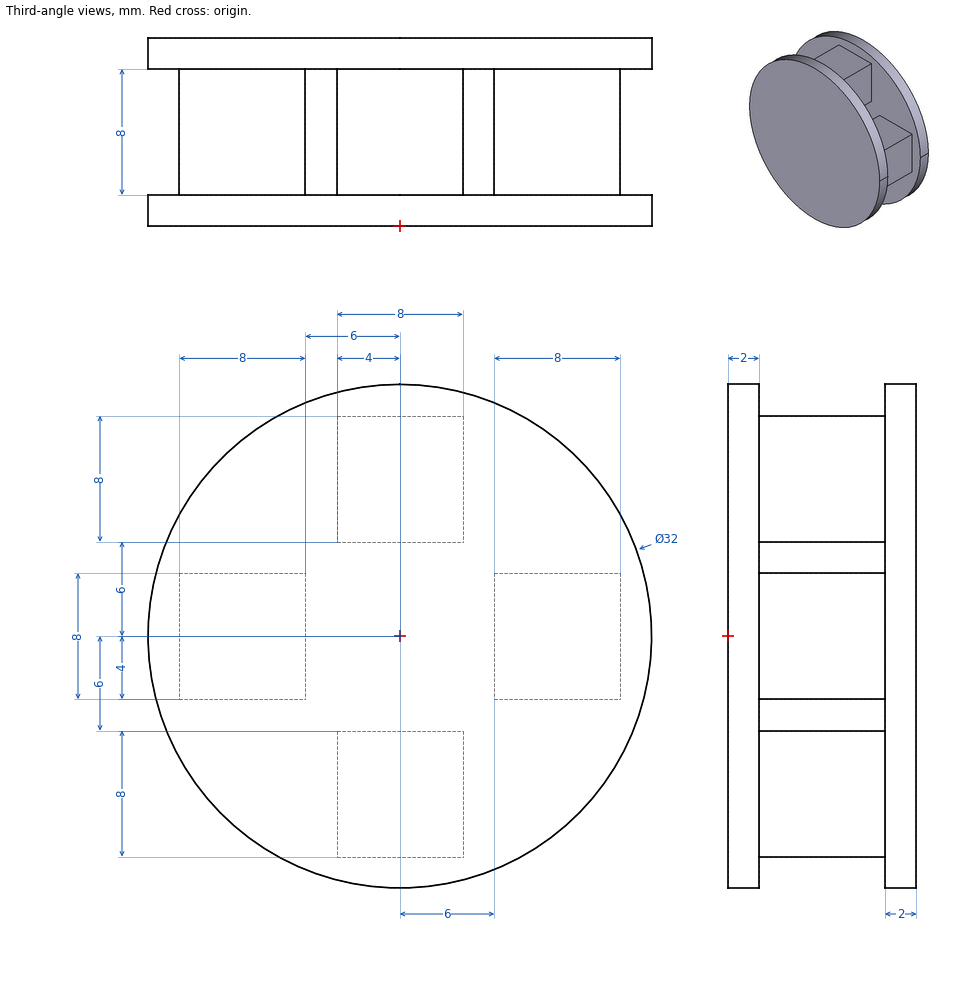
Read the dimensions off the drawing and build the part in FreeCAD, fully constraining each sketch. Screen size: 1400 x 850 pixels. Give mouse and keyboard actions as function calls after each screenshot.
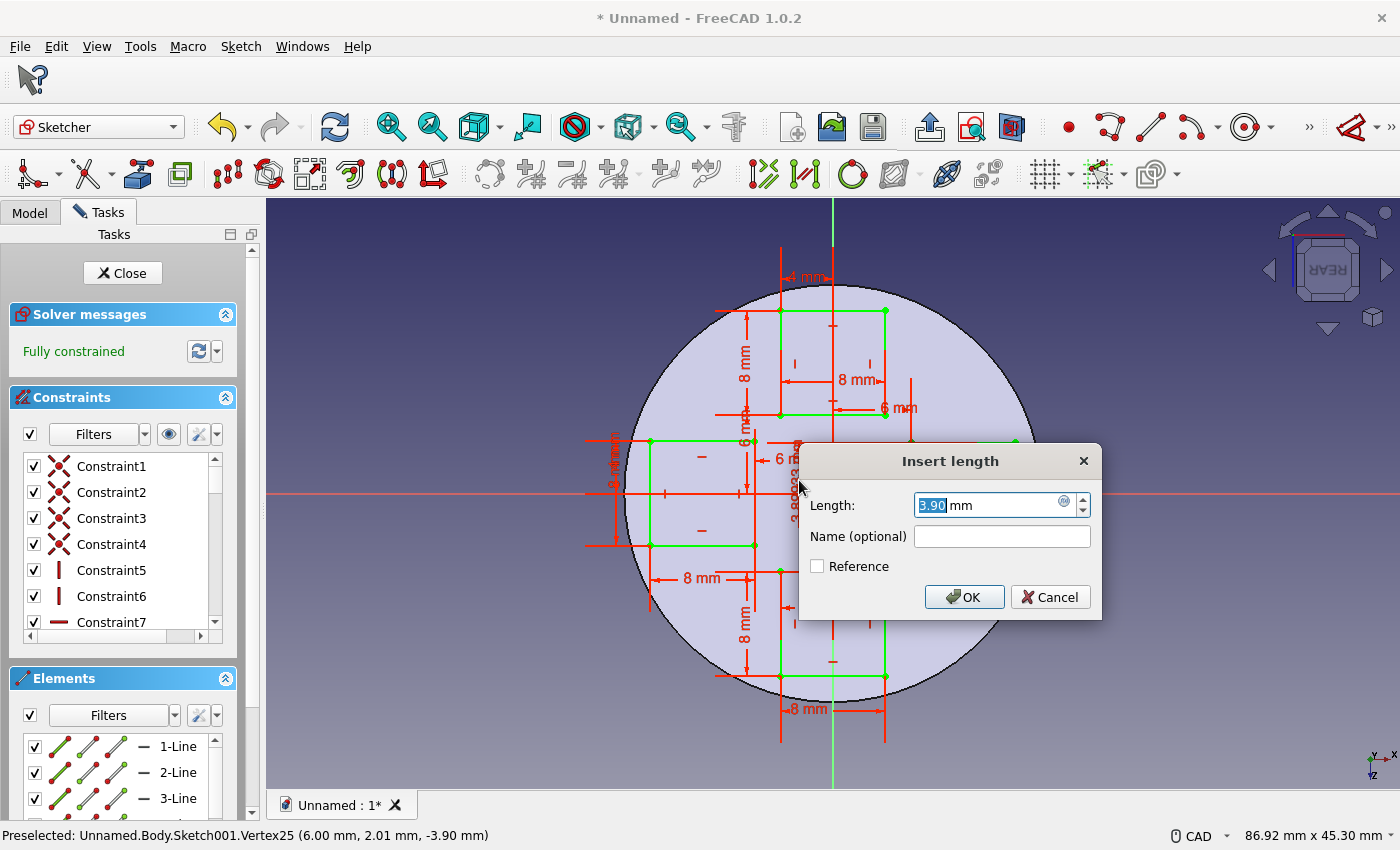
text(4)
key(Return)
key(Escape)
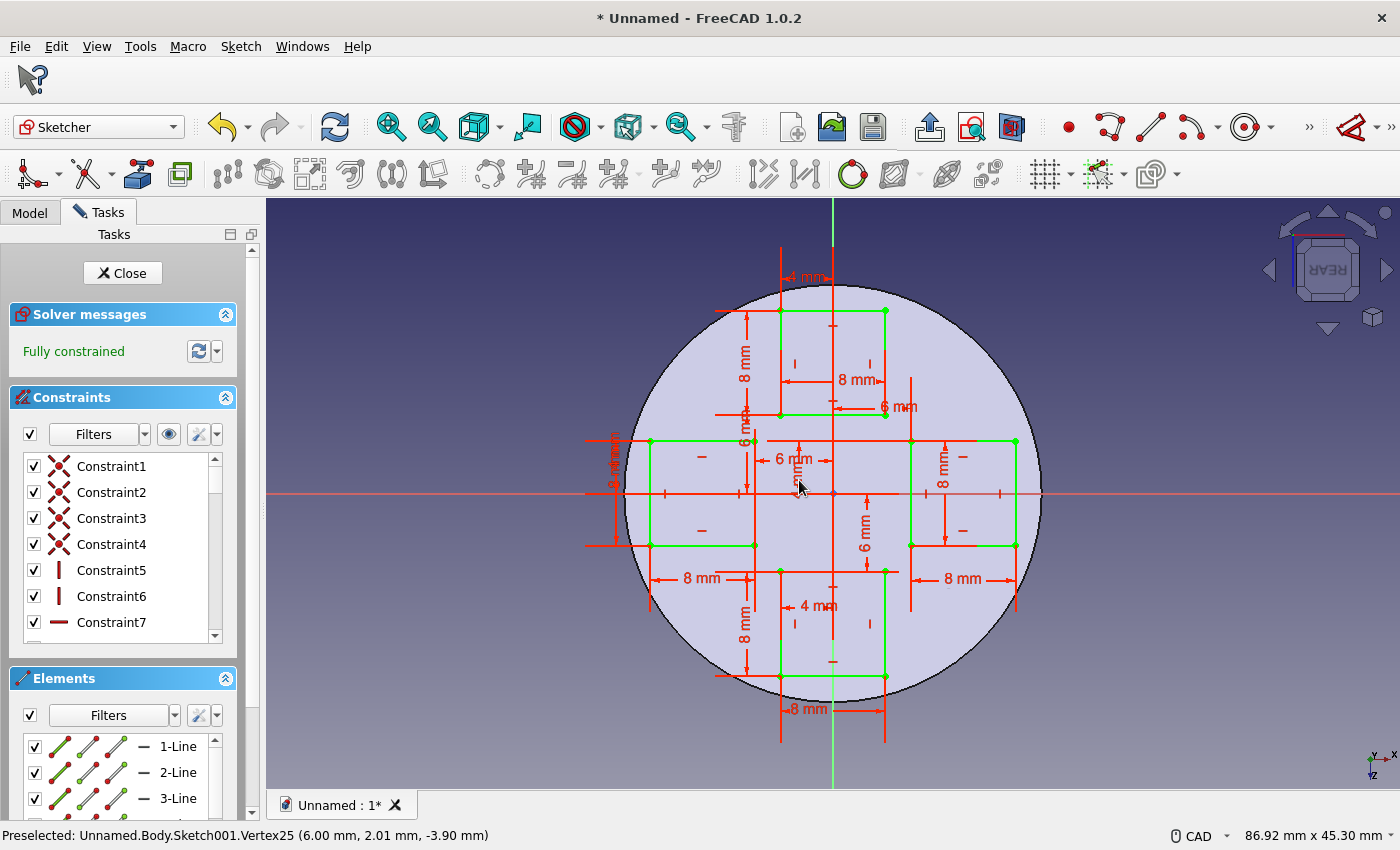
click(123, 273)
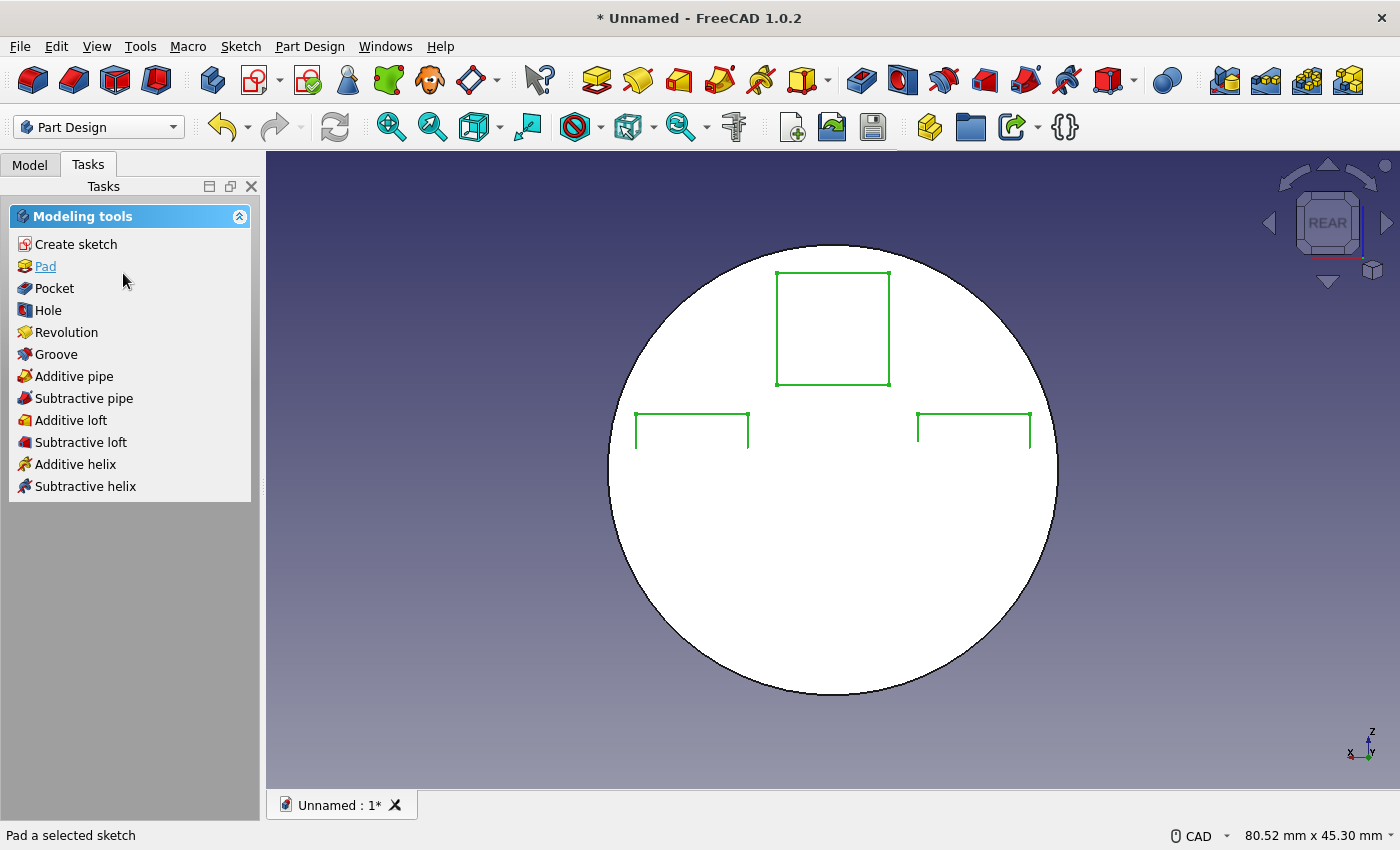
click(597, 80)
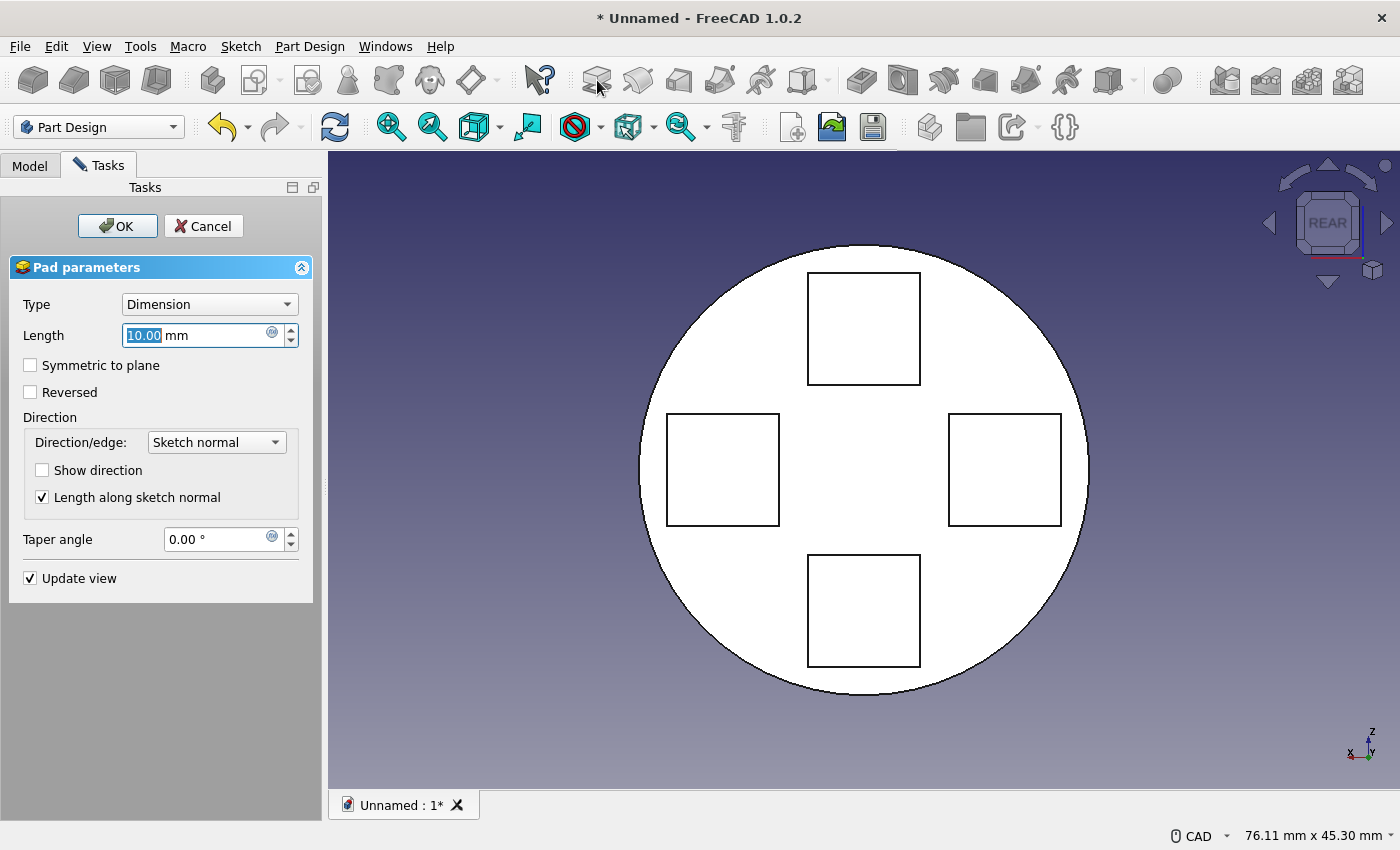
text(8)
key(Tab)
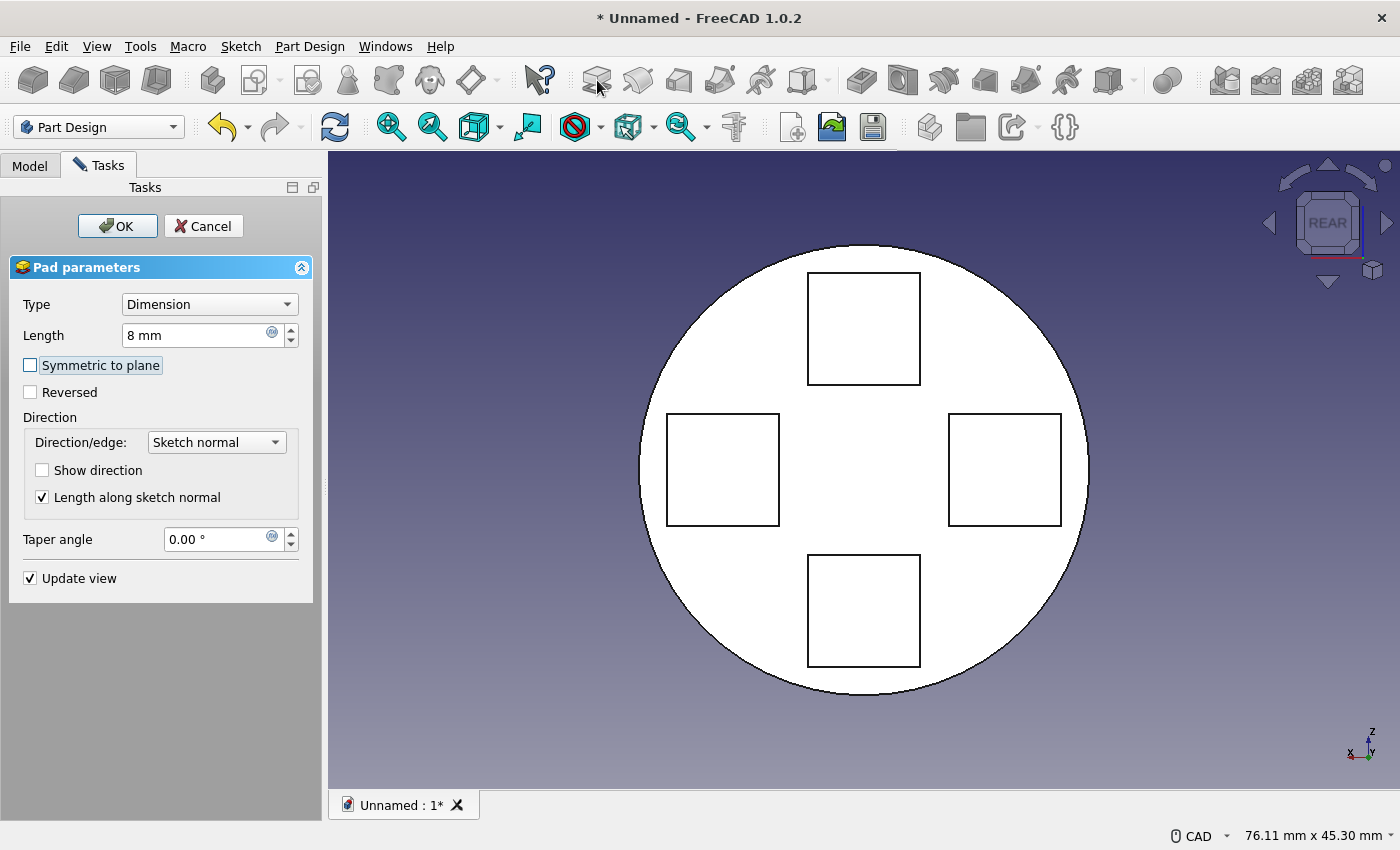
click(118, 226)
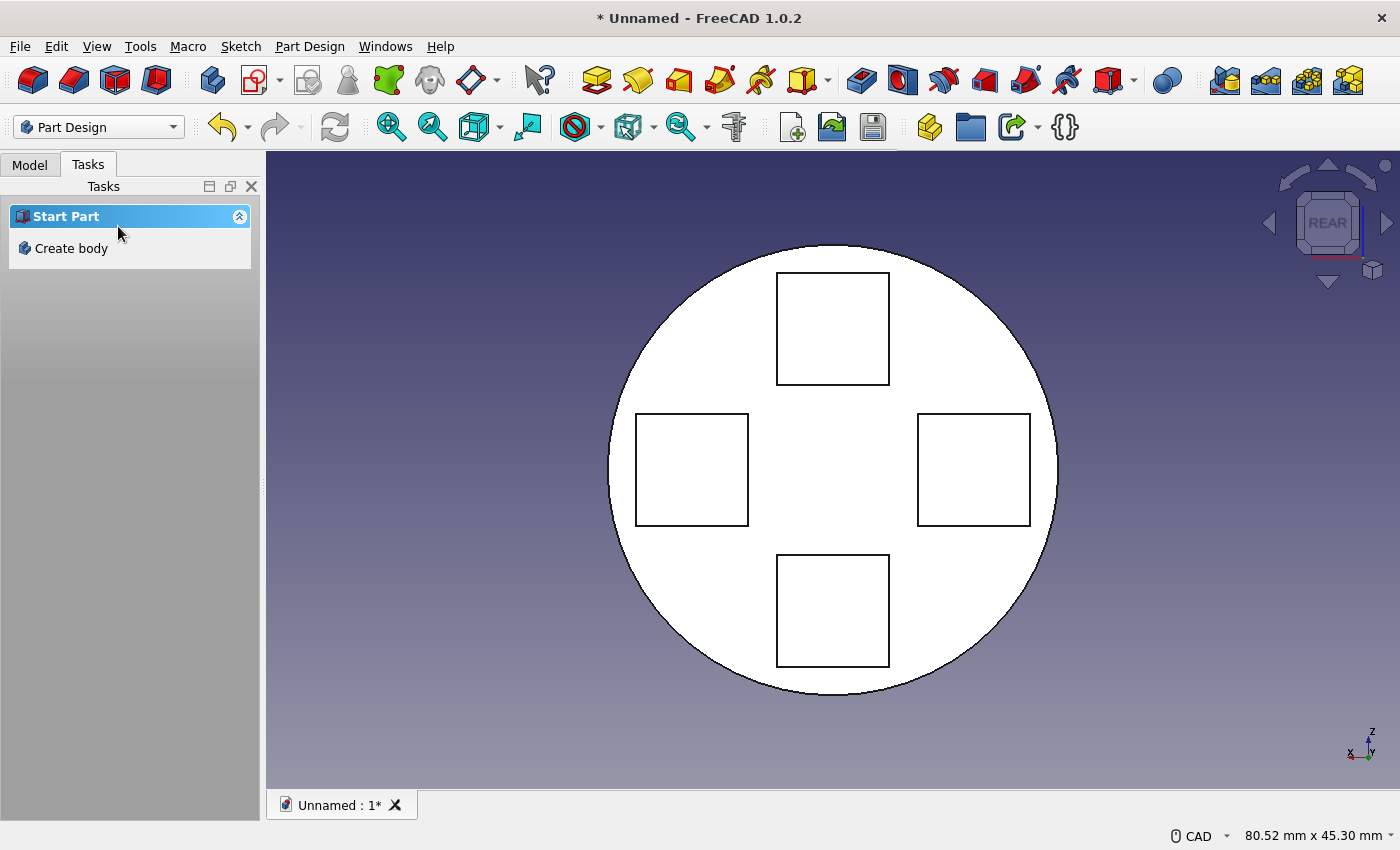
click(692, 469)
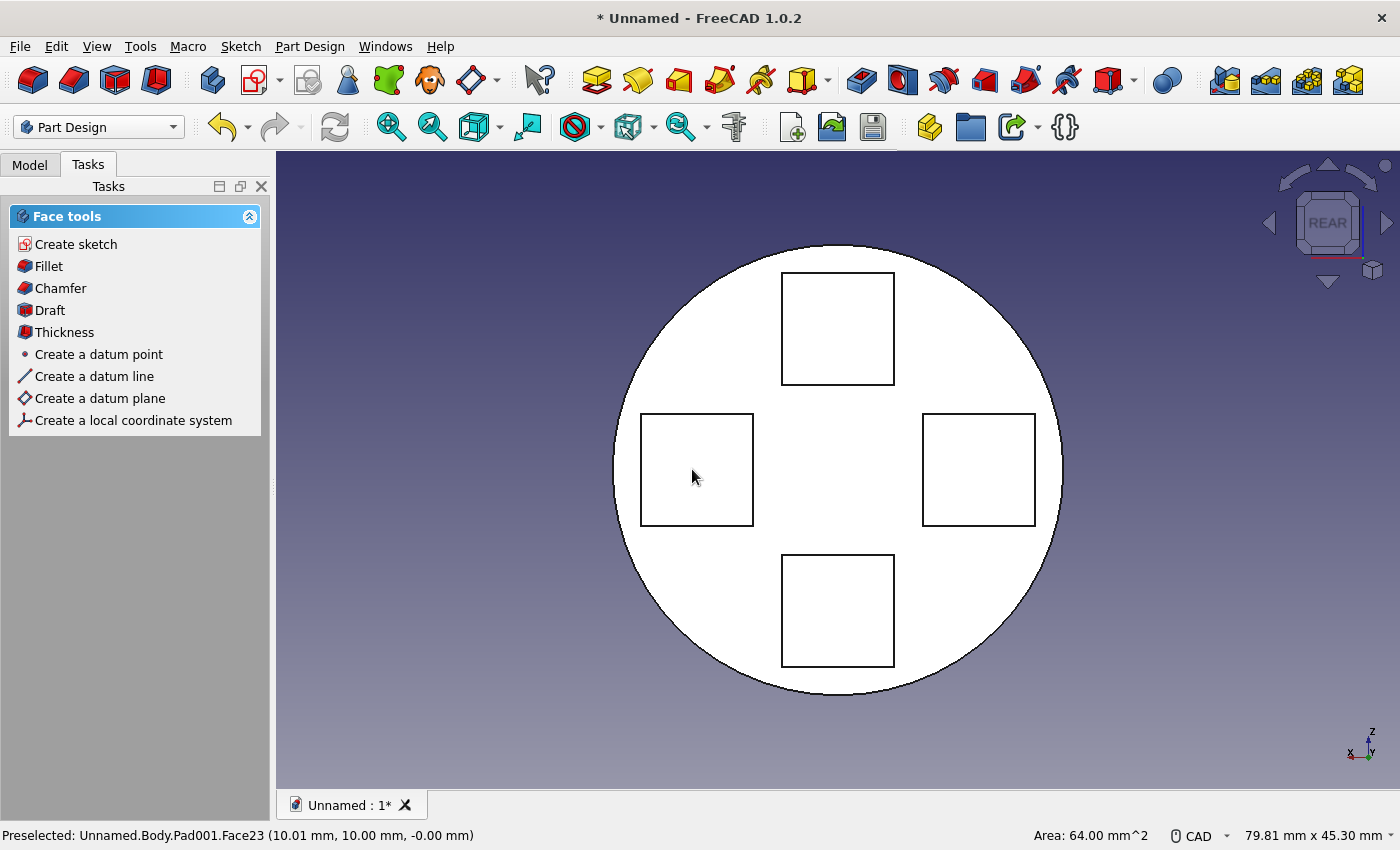
click(254, 80)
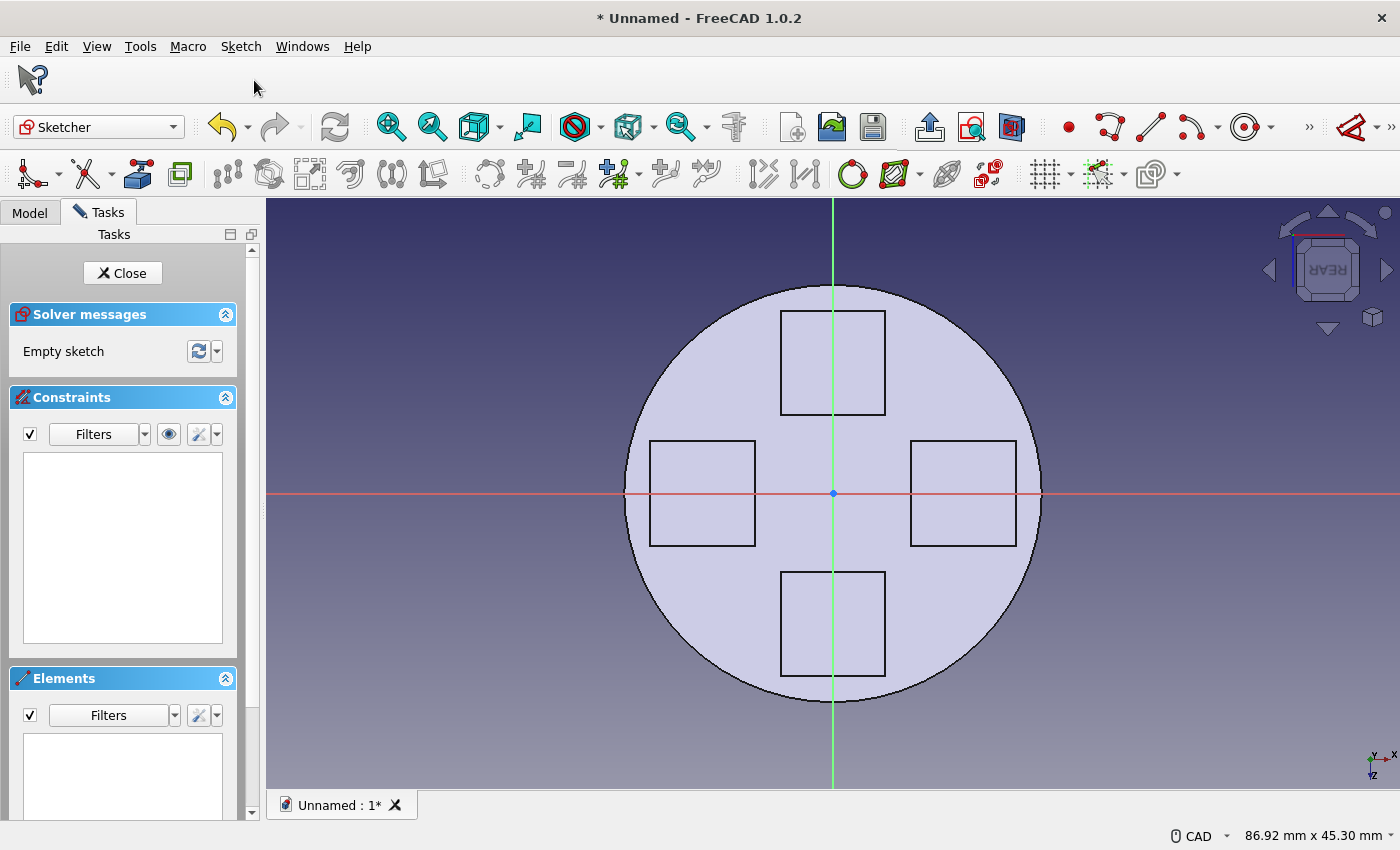
key(g)
key(c)